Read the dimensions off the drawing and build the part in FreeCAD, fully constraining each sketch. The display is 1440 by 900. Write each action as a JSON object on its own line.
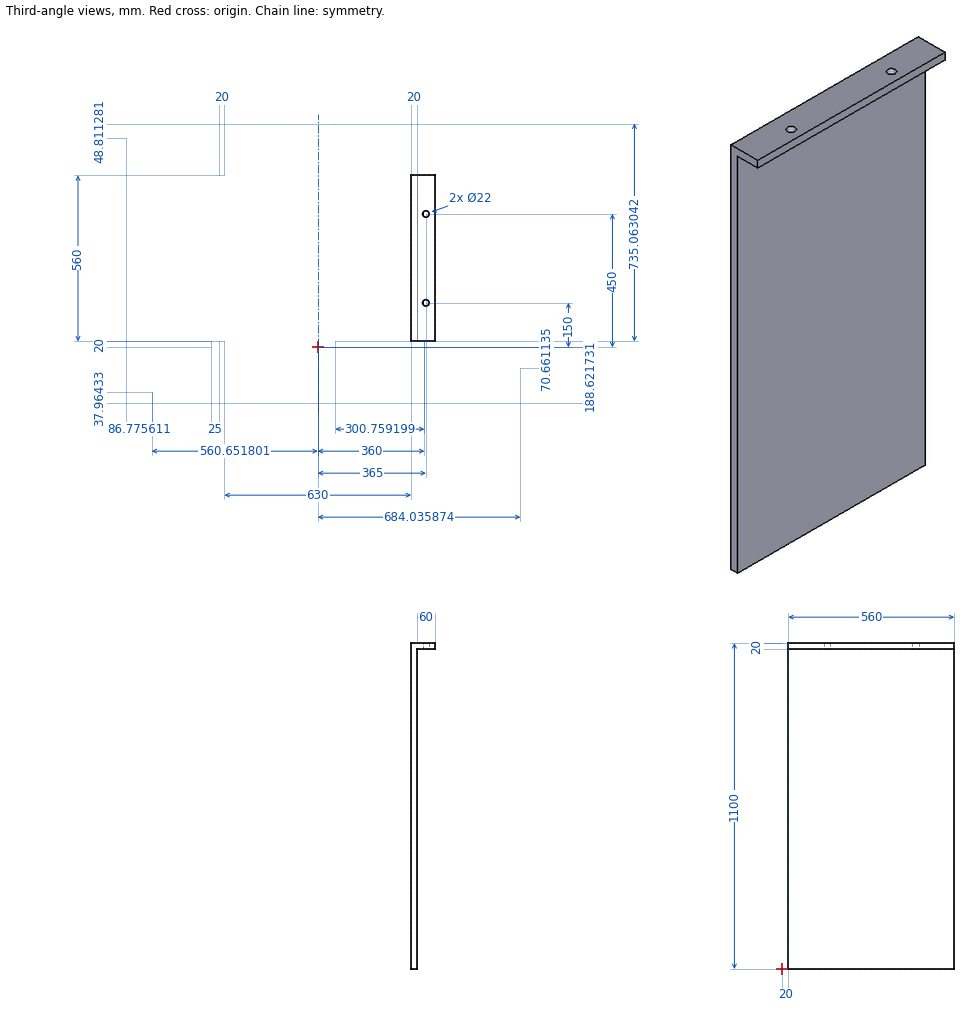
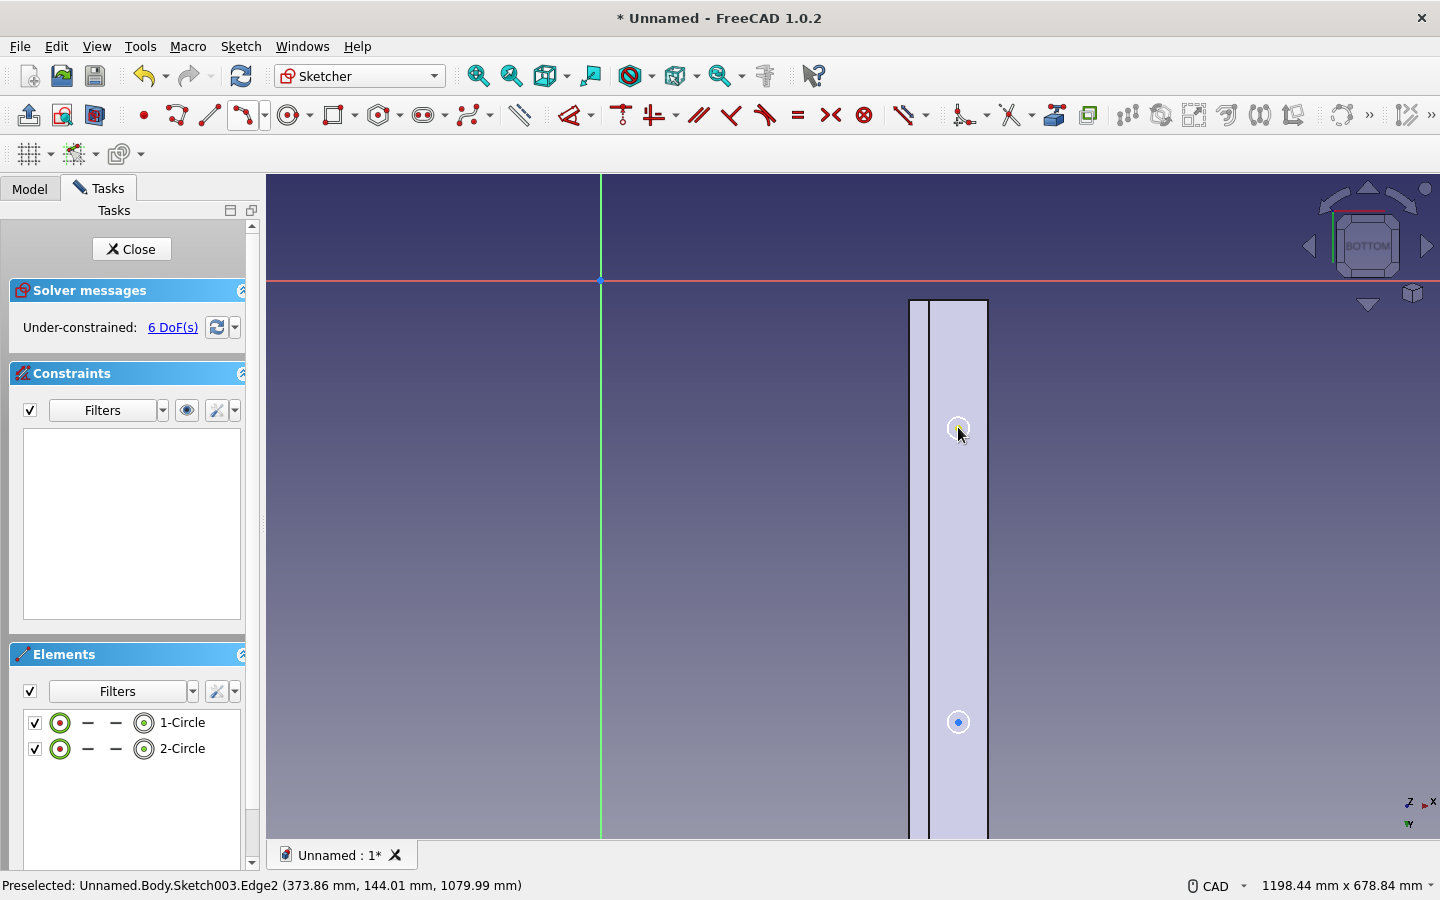
{"action": "scroll", "coordinate": [966, 714], "scroll_direction": "up", "scroll_amount": 2}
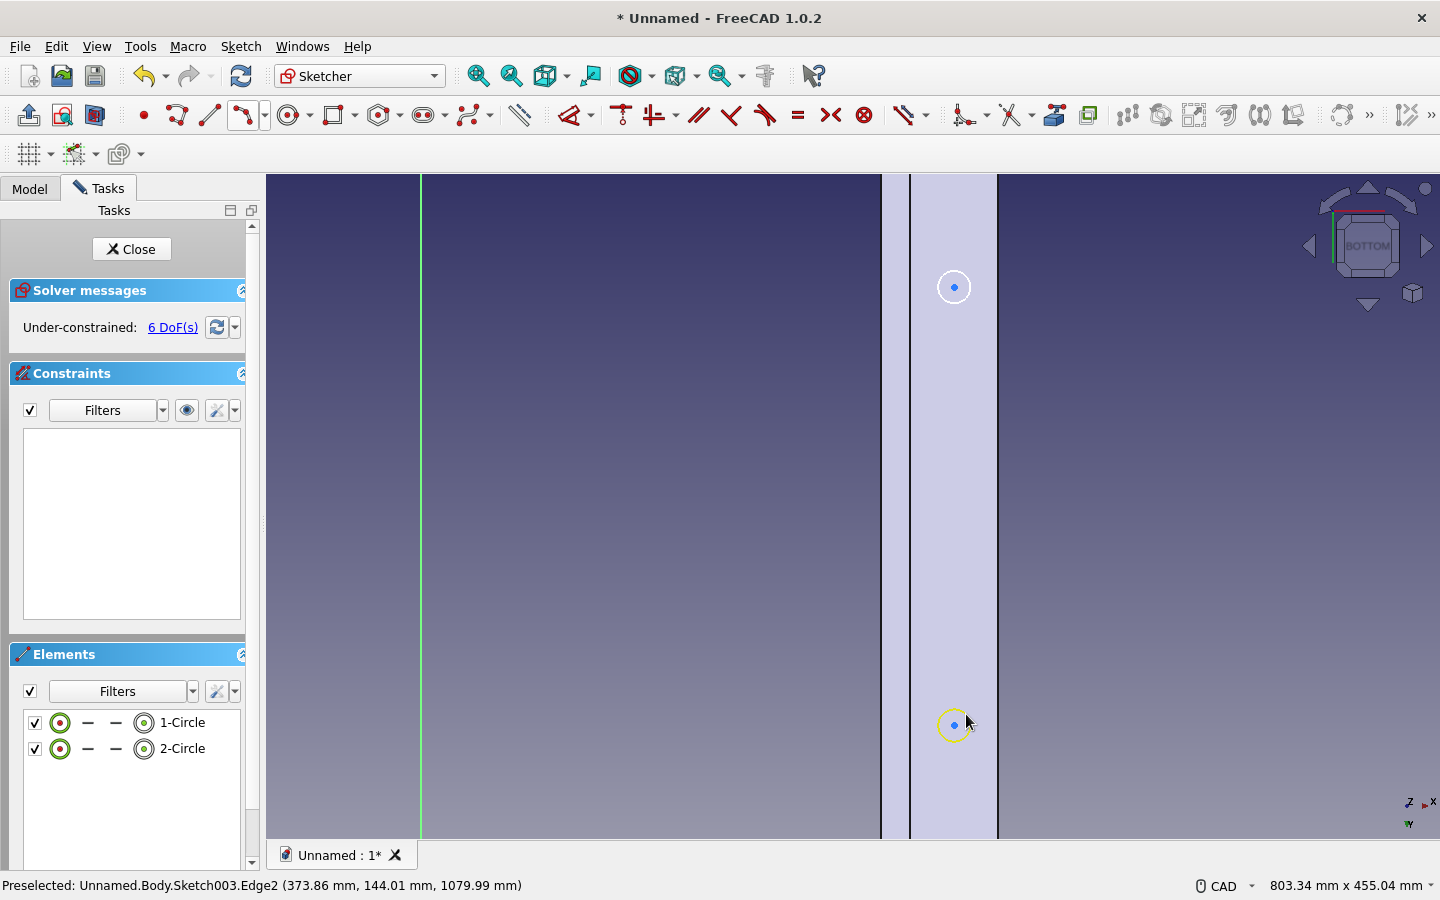
{"action": "left_click", "coordinate": [966, 714]}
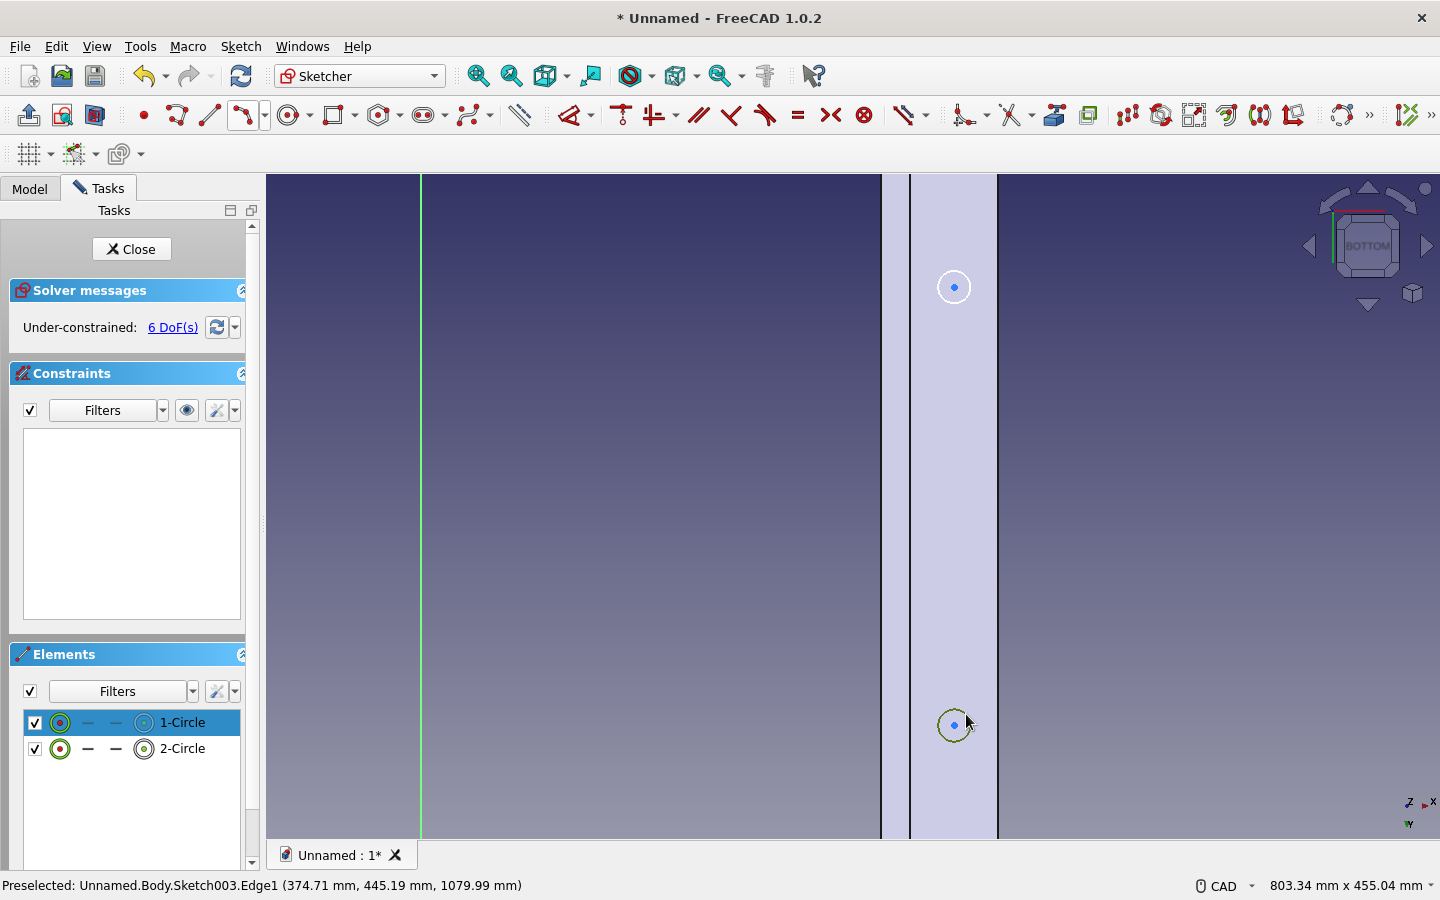
{"action": "left_click", "coordinate": [966, 276]}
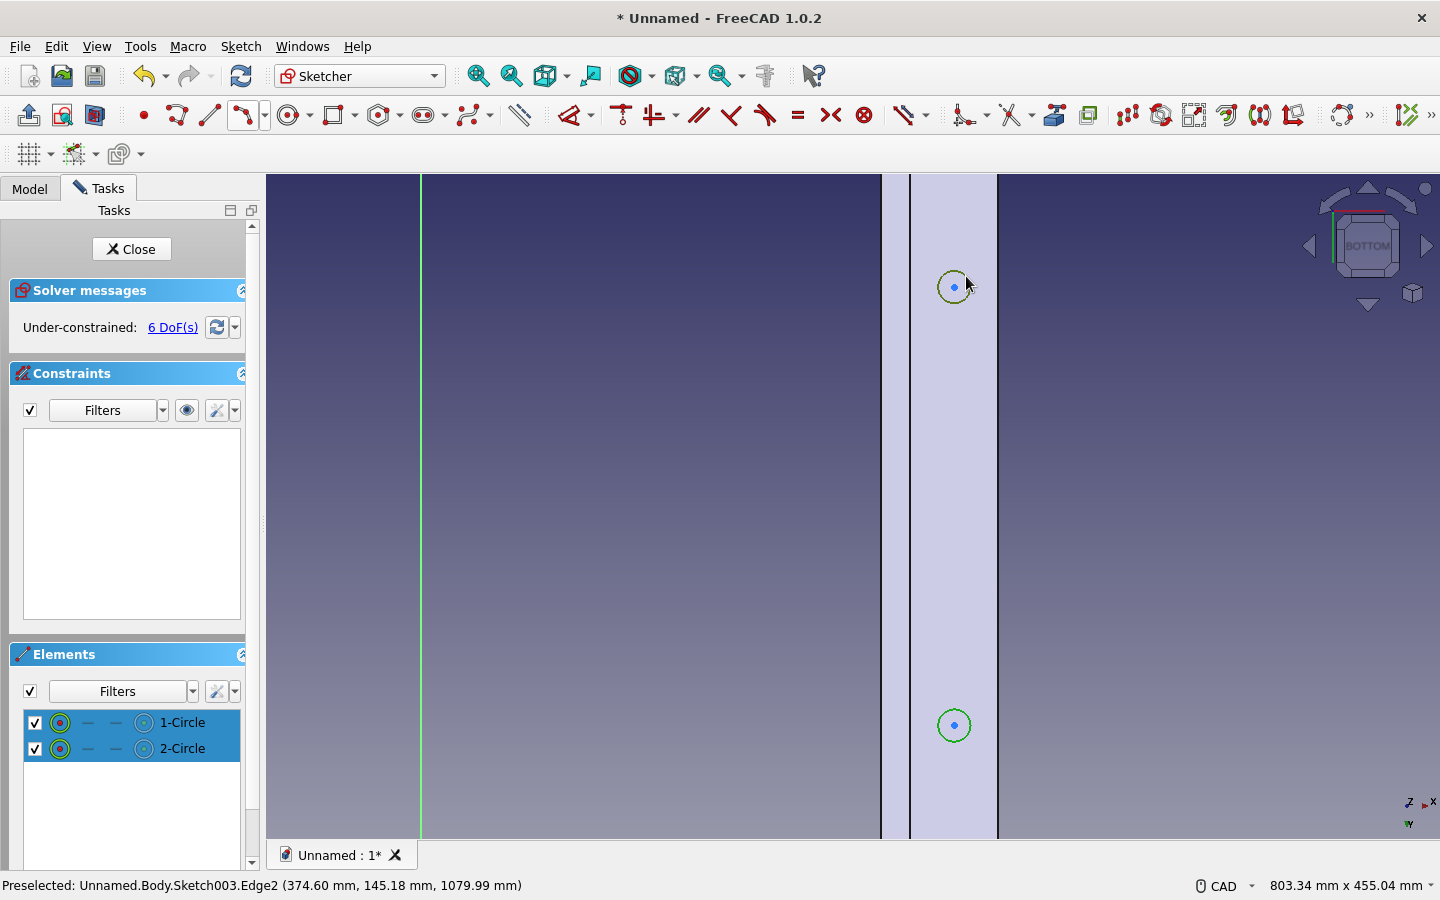
{"action": "left_click", "coordinate": [798, 116]}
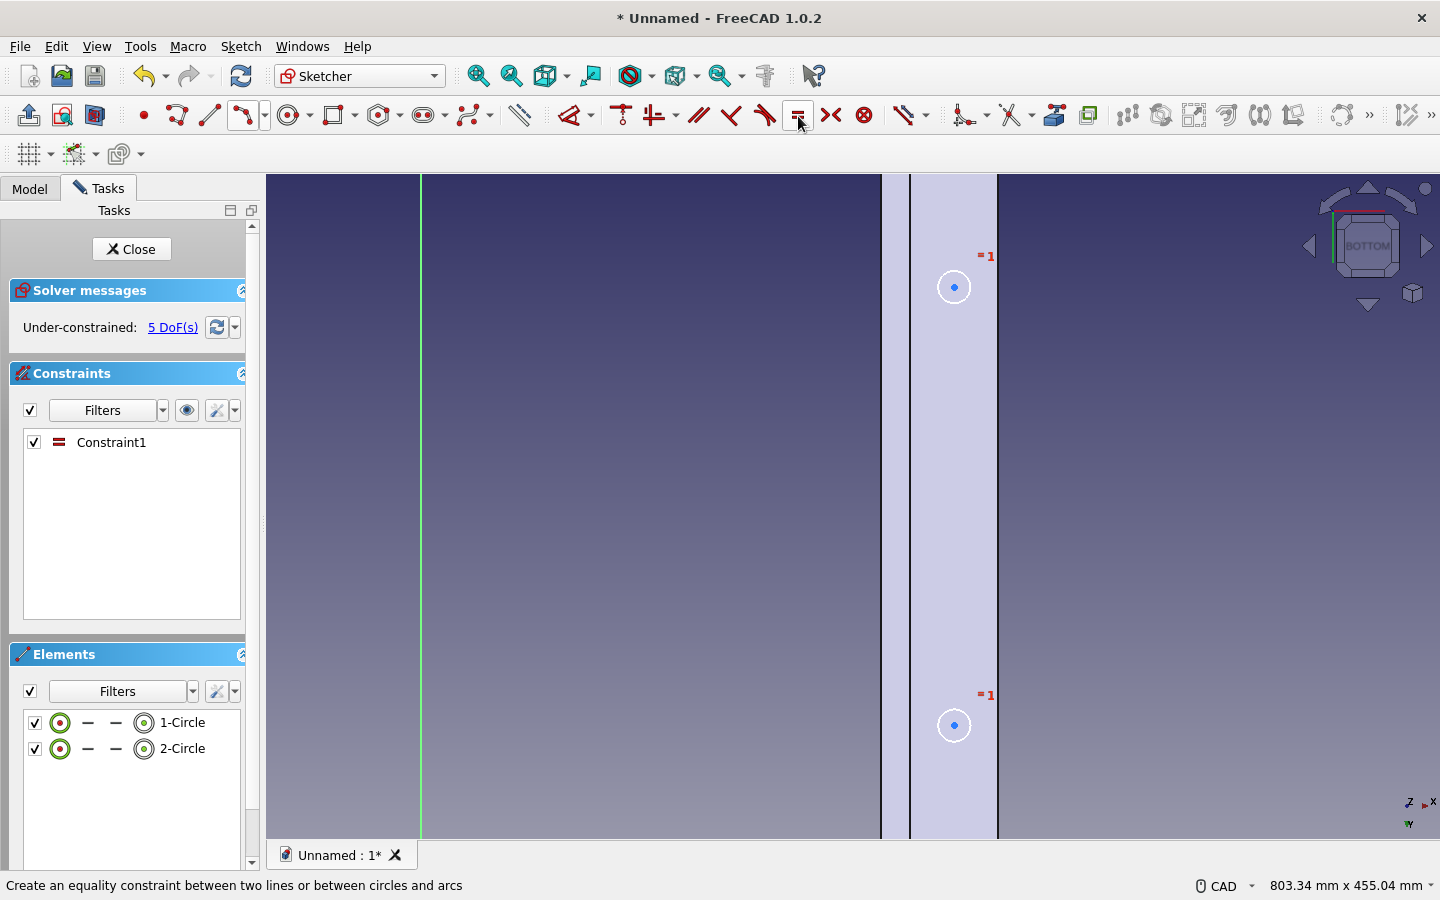
{"action": "left_click", "coordinate": [954, 726]}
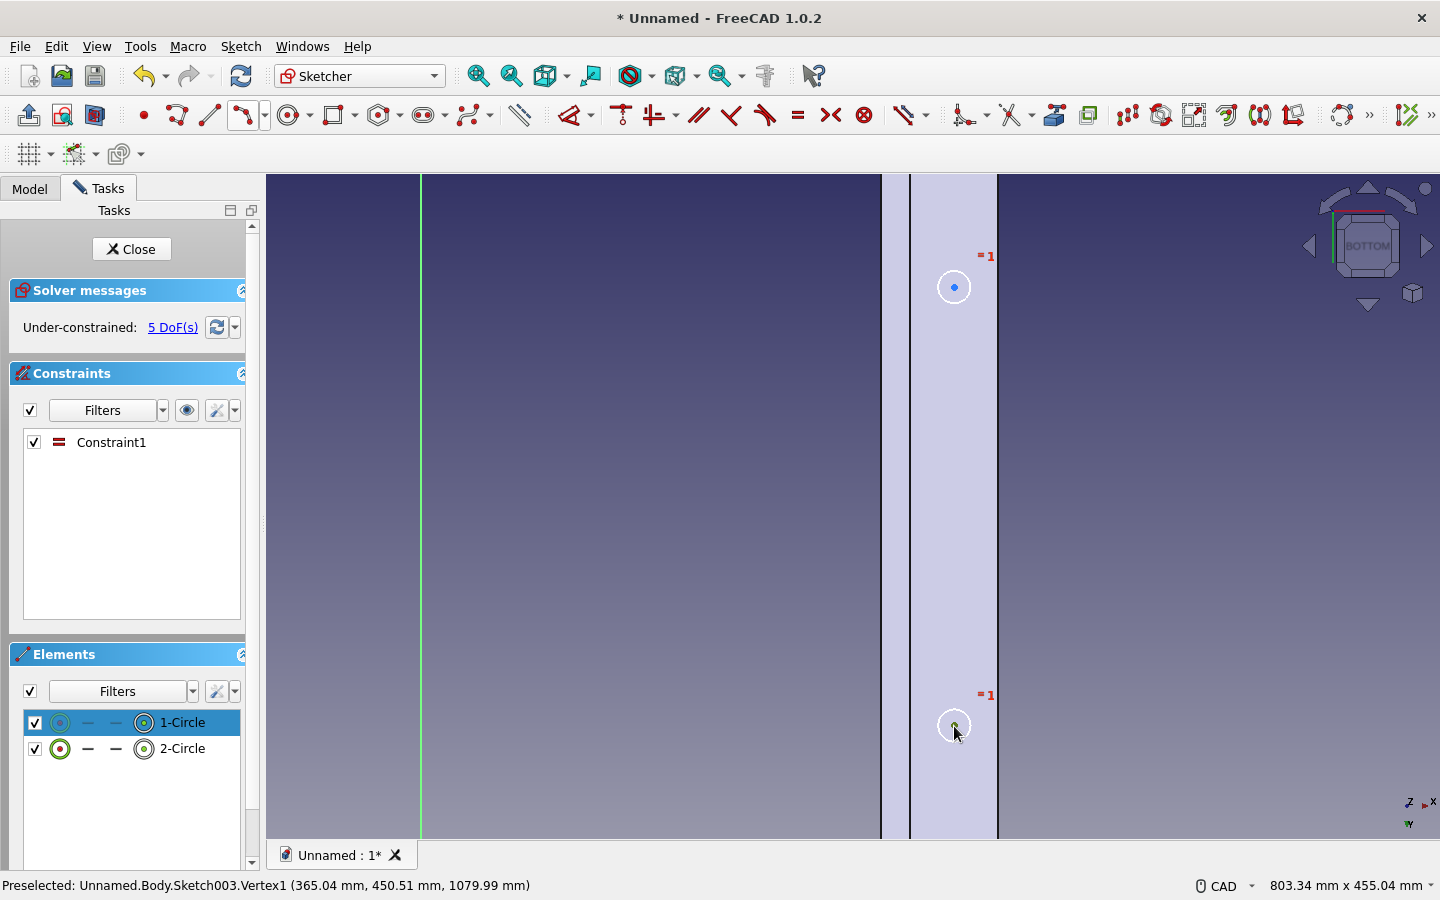
{"action": "left_click", "coordinate": [954, 287]}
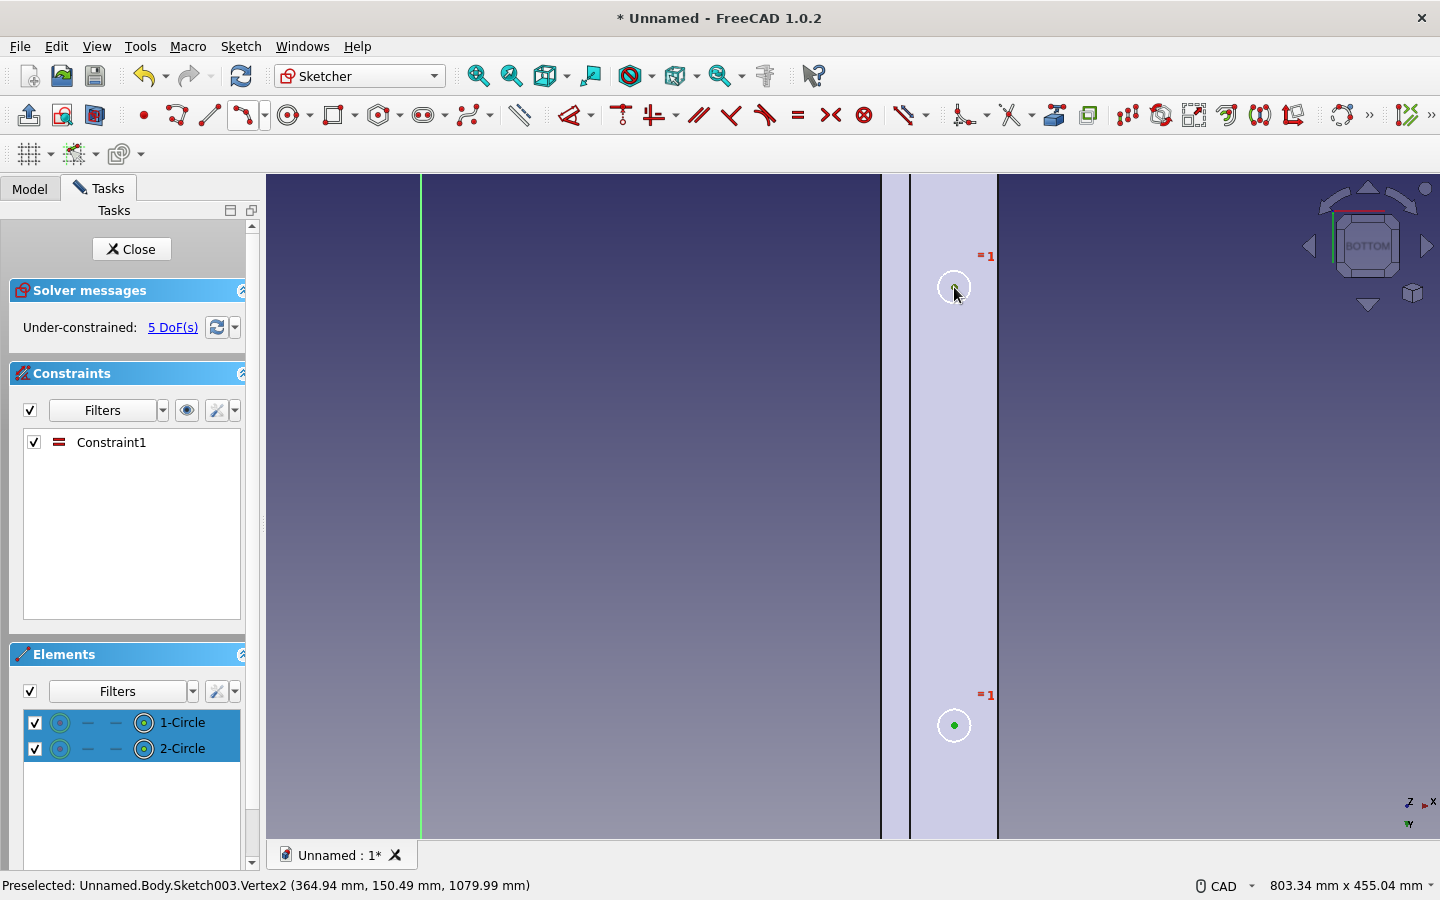
{"action": "key", "text": "v"}